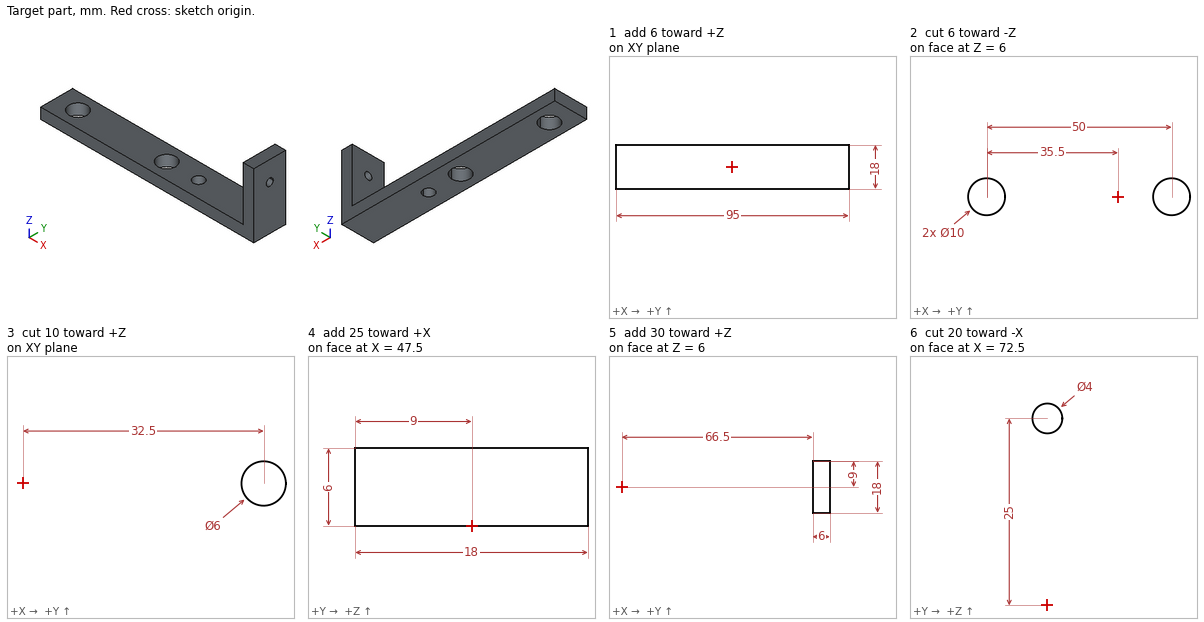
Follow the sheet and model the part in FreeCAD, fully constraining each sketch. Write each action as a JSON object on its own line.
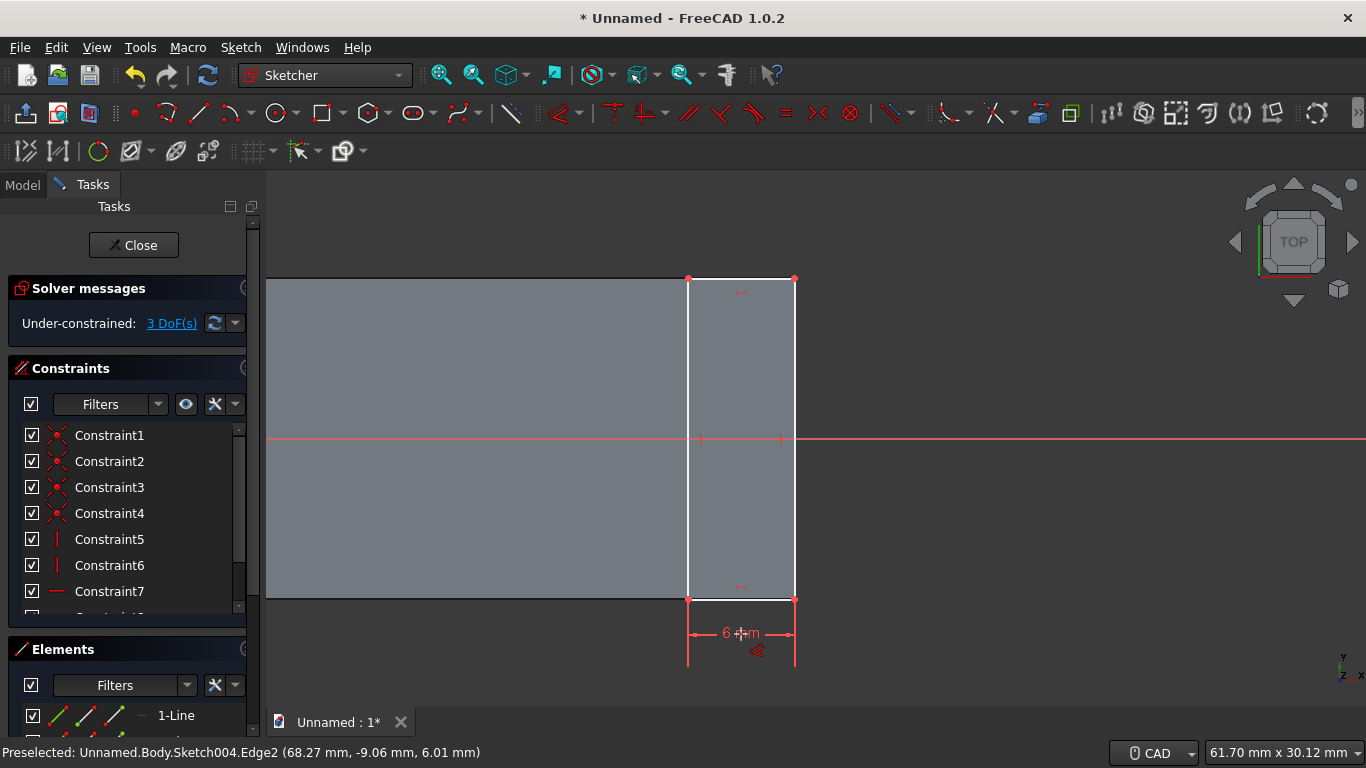
{"action": "left_click", "coordinate": [688, 375]}
{"action": "left_click", "coordinate": [654, 366]}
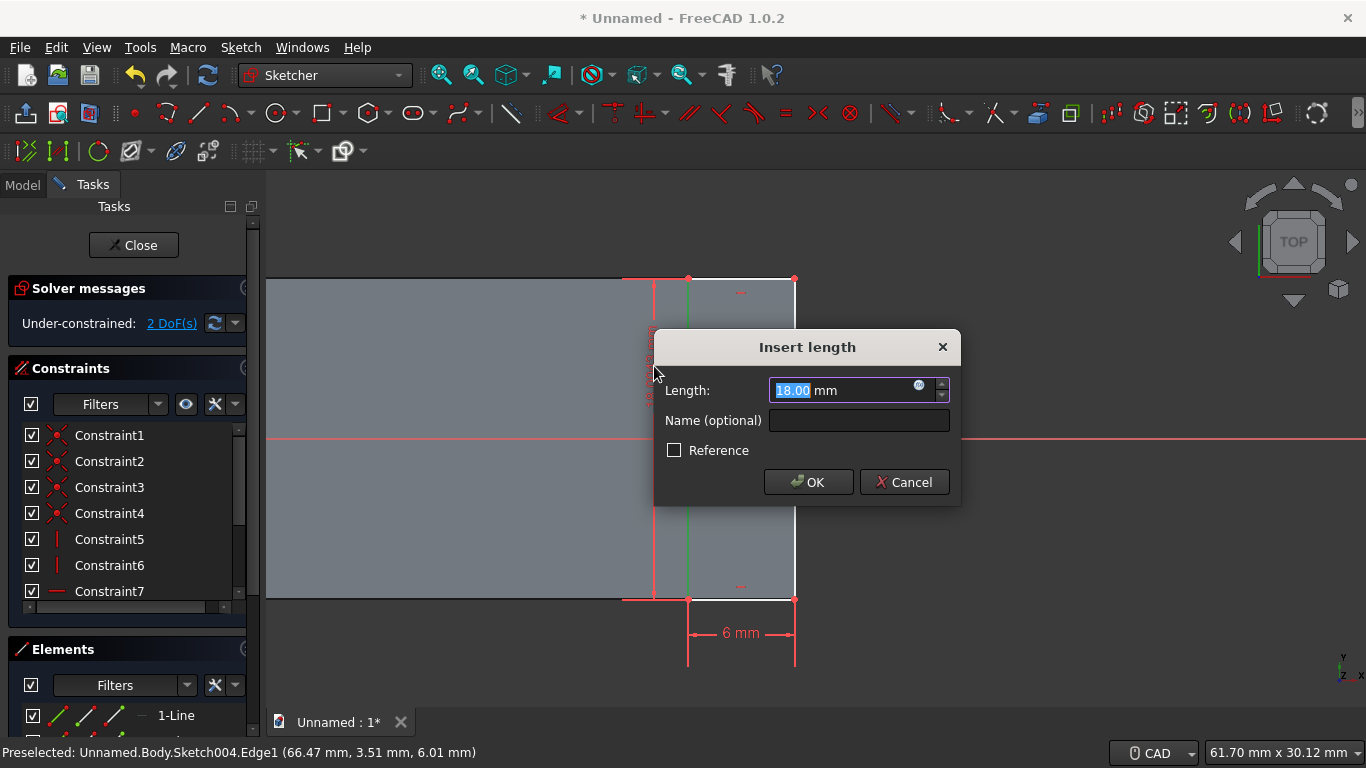
{"action": "type", "text": "18"}
{"action": "key", "text": "Return"}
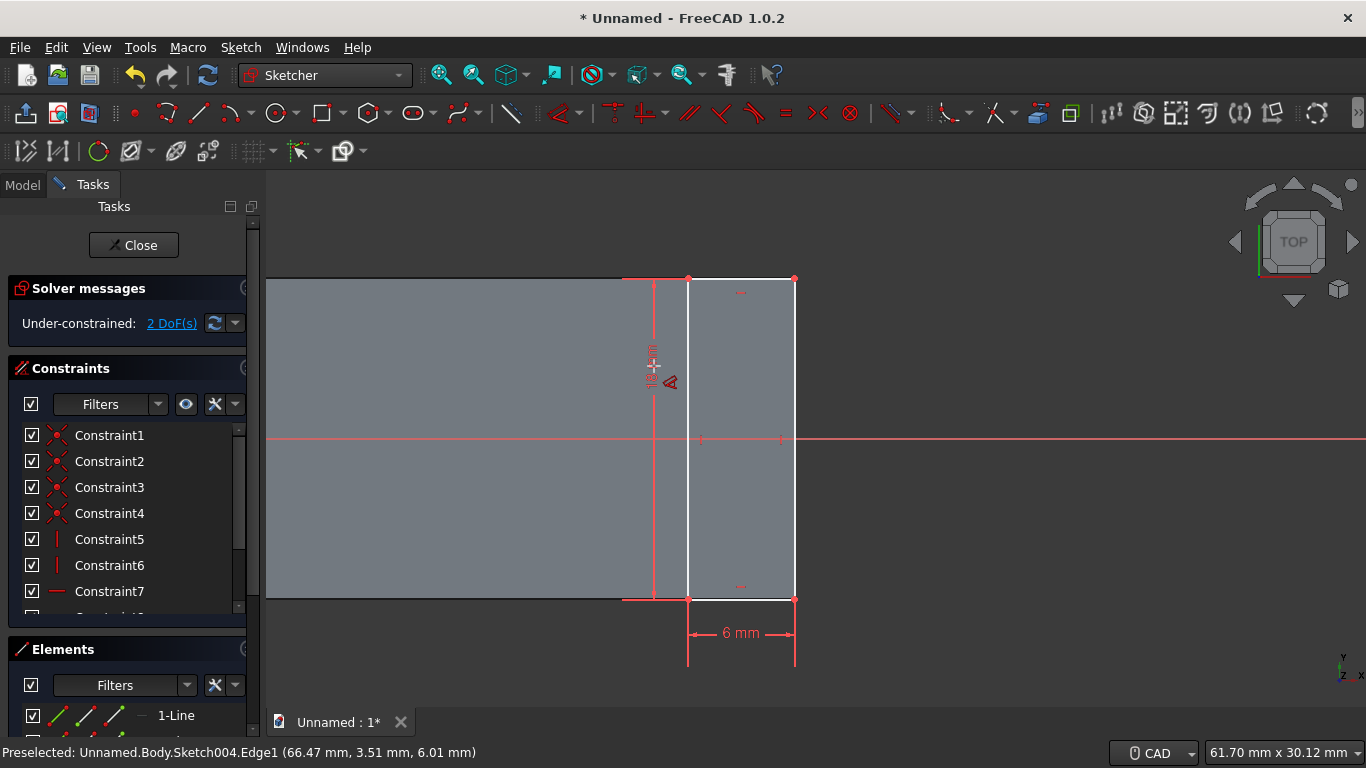
{"action": "left_click", "coordinate": [688, 279]}
{"action": "left_click", "coordinate": [722, 322]}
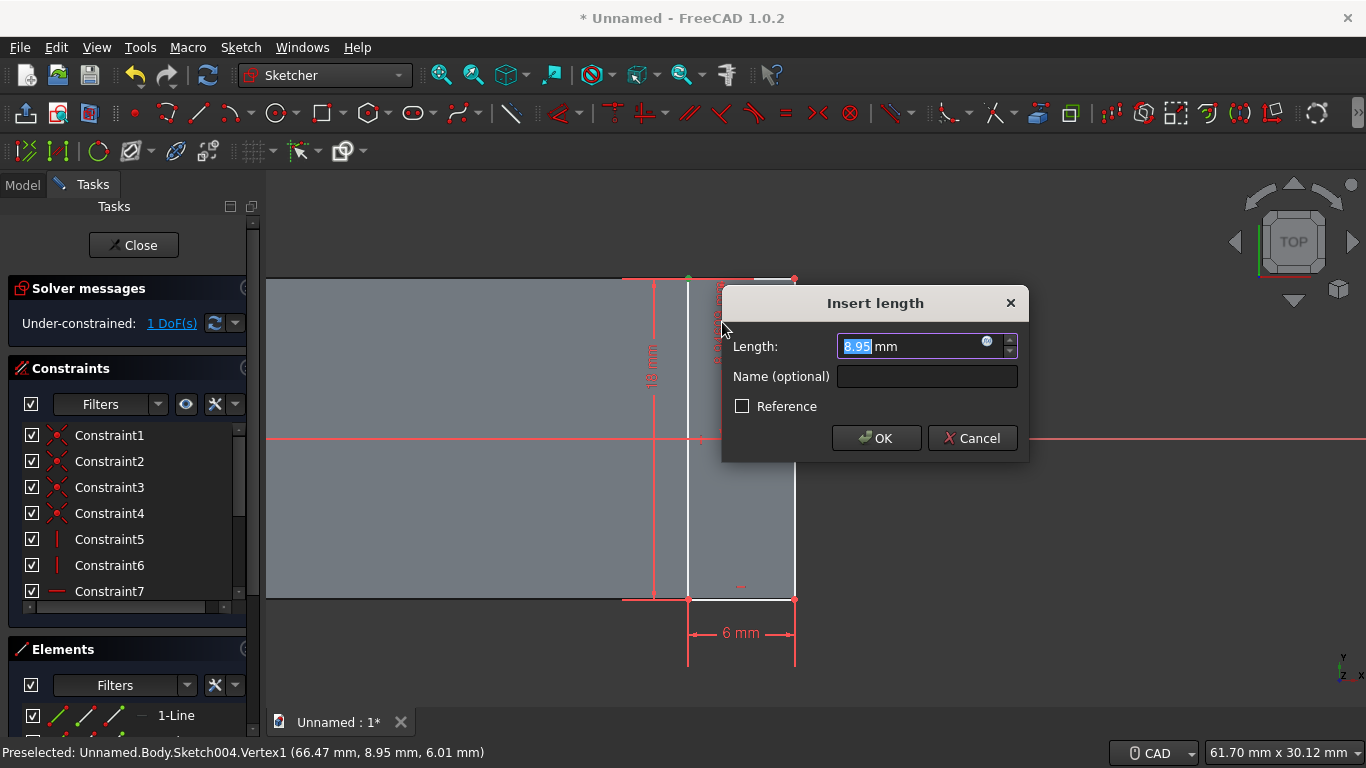
{"action": "type", "text": "9"}
{"action": "key", "text": "Return"}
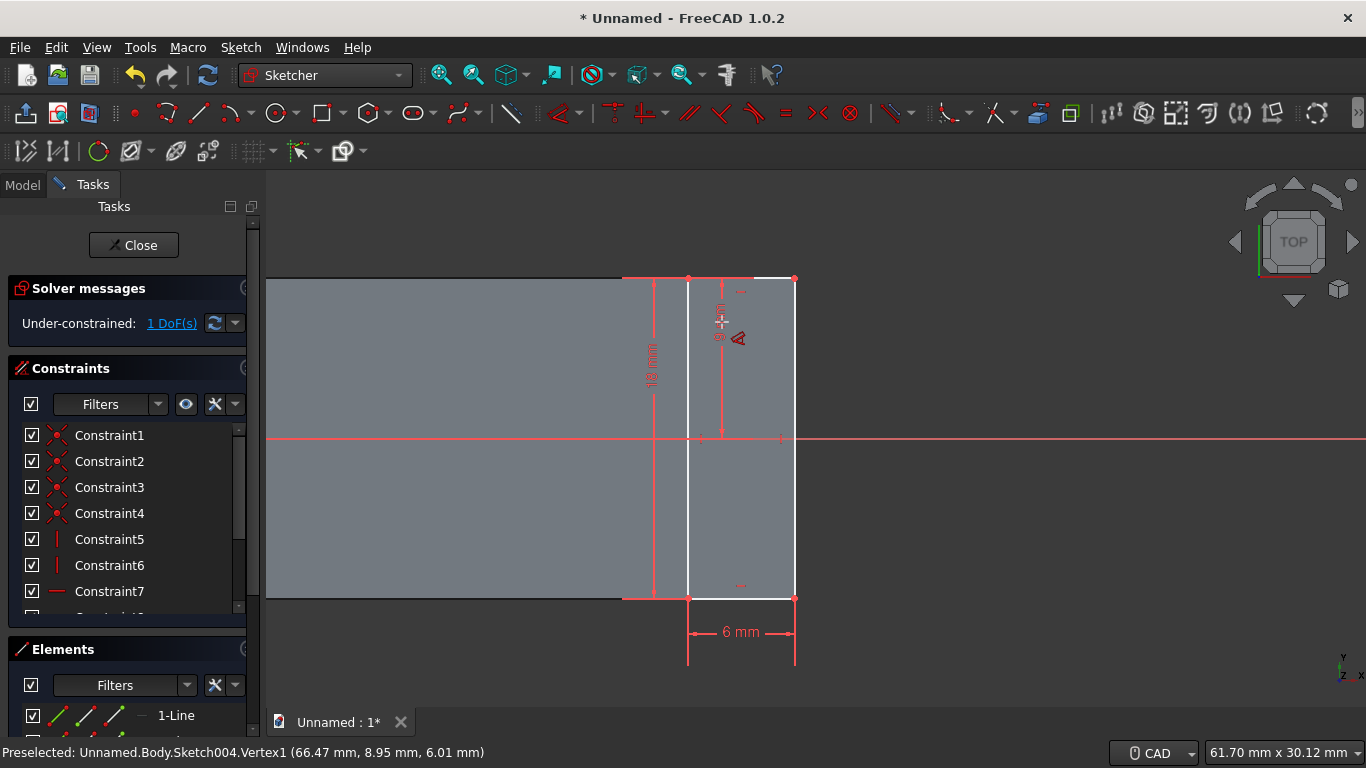
{"action": "left_click", "coordinate": [688, 278]}
{"action": "left_click", "coordinate": [491, 244]}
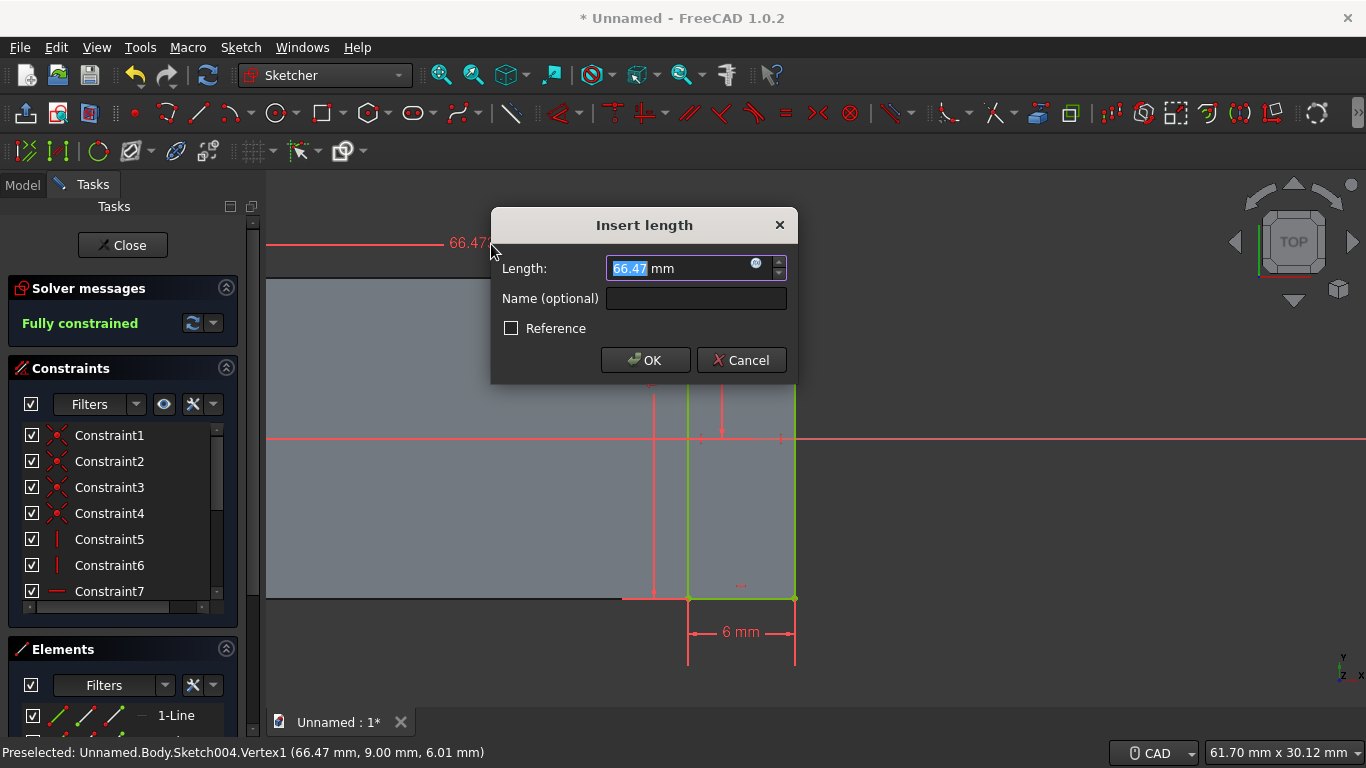
{"action": "type", "text": "66.5"}
{"action": "key", "text": "Return"}
{"action": "key", "text": "Escape"}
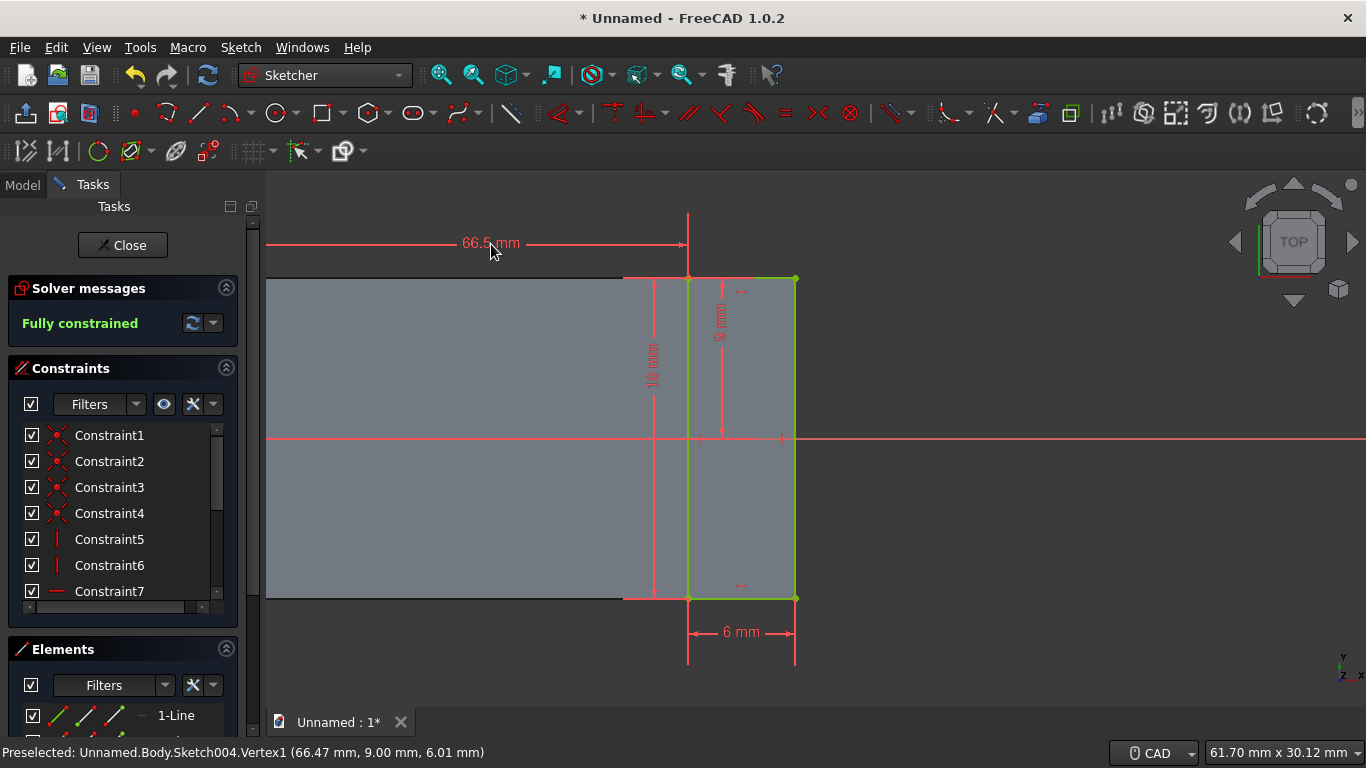
{"action": "left_click", "coordinate": [123, 245]}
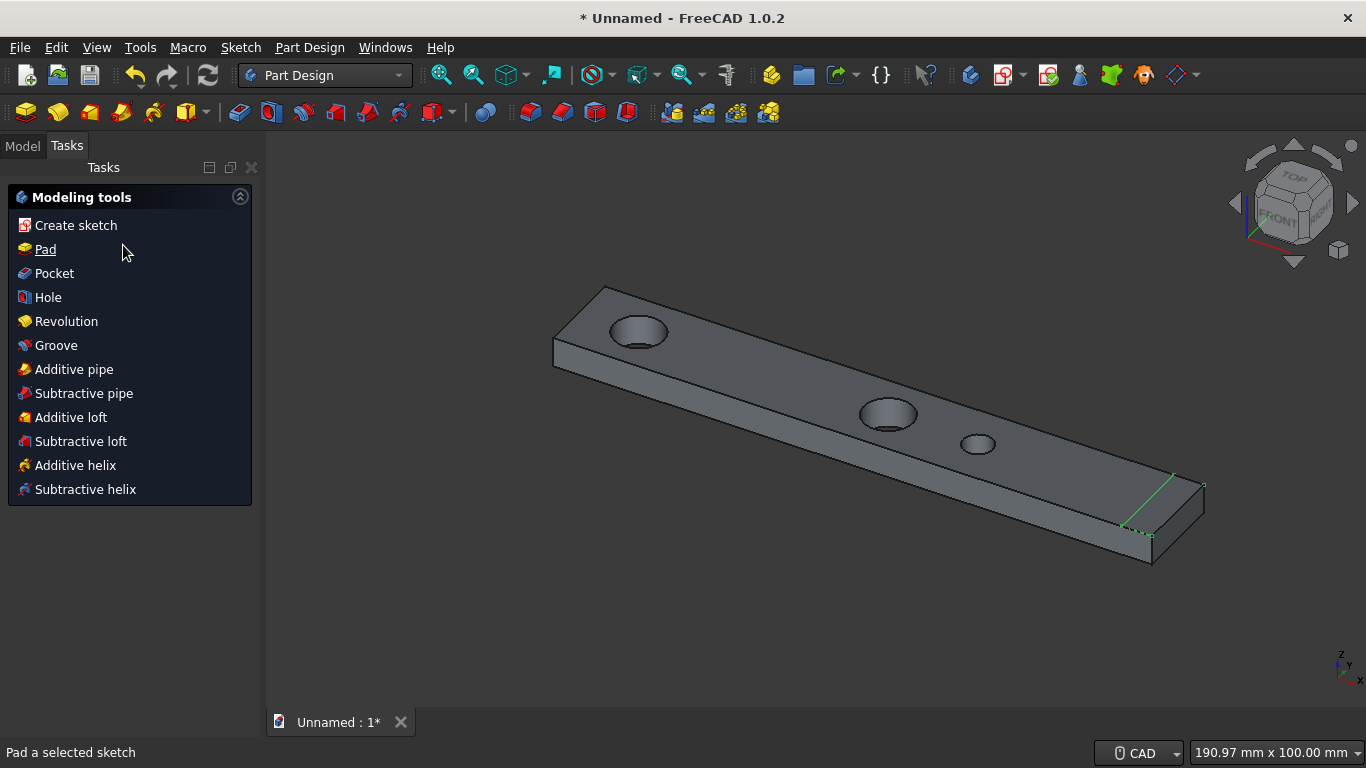
{"action": "left_click", "coordinate": [26, 112]}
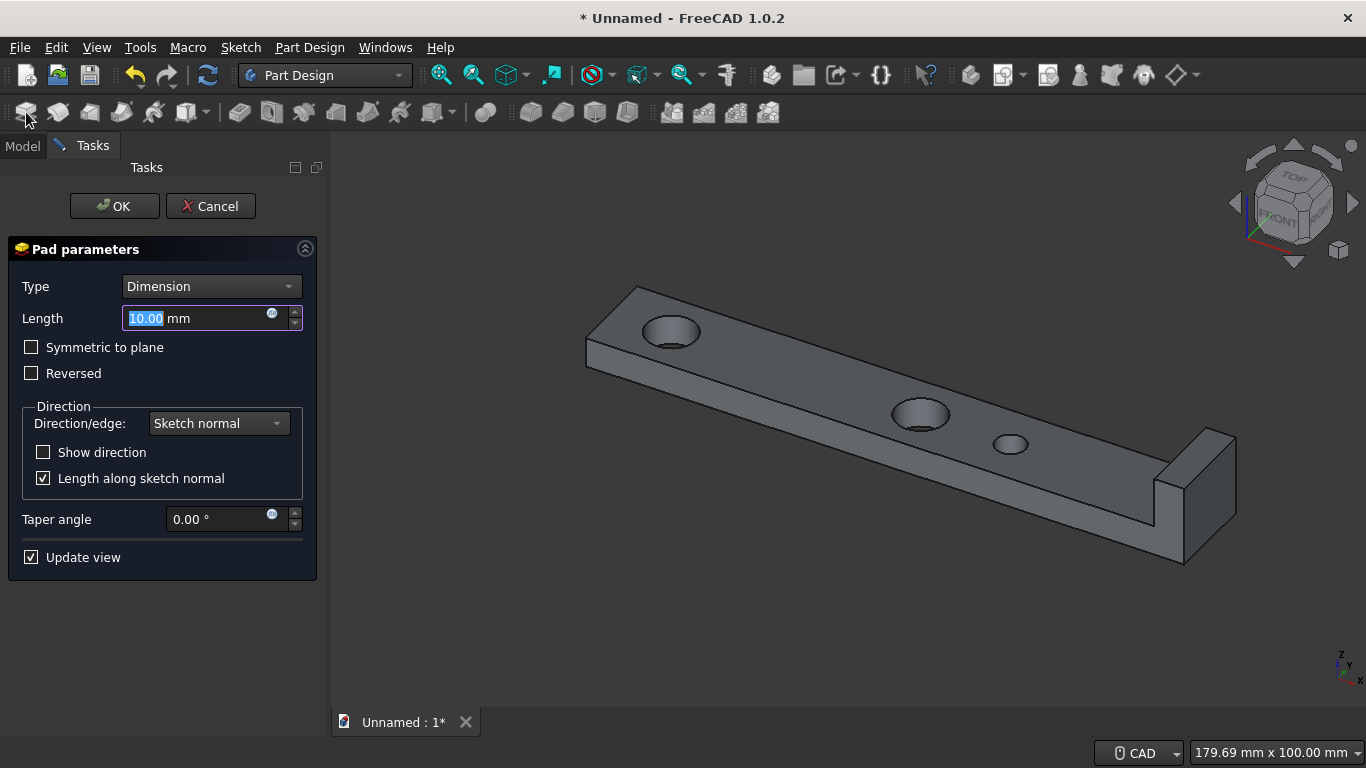
{"action": "type", "text": "30"}
{"action": "key", "text": "Tab"}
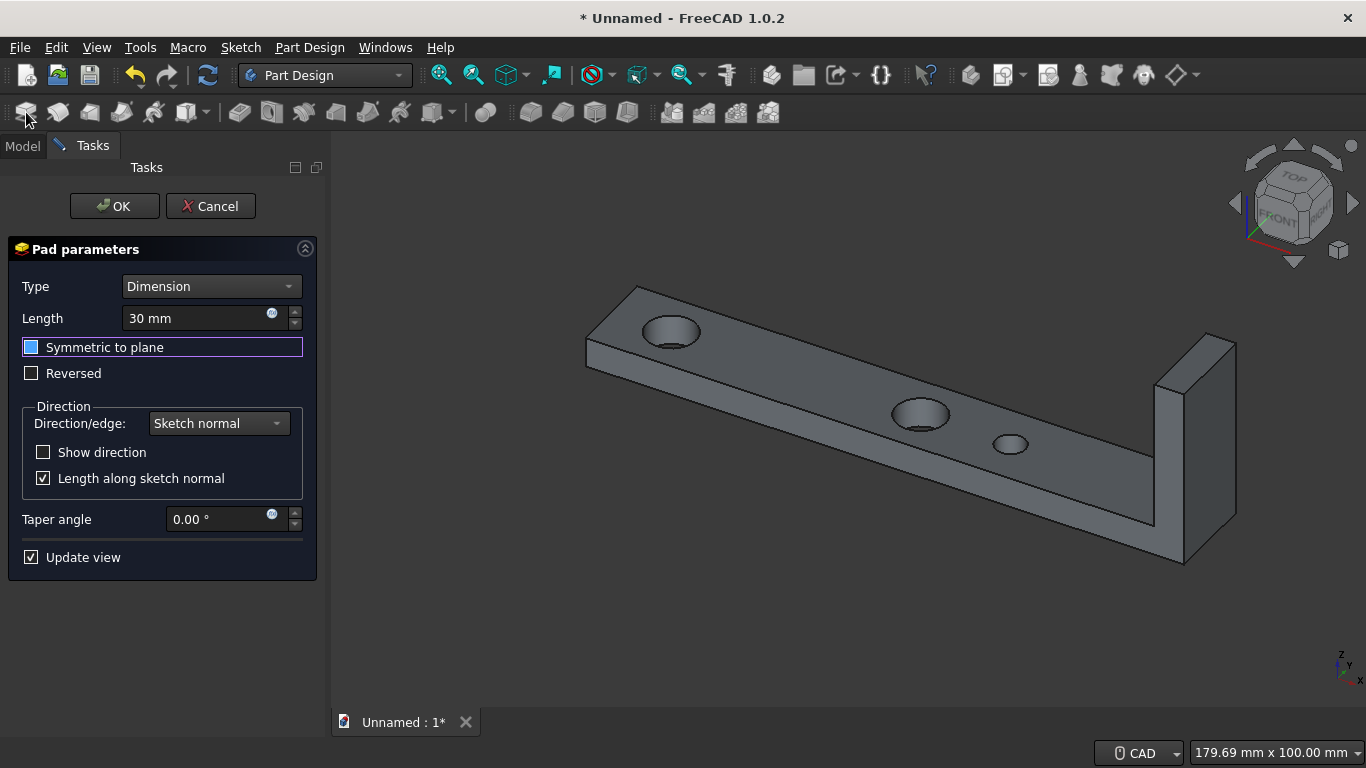
{"action": "left_click", "coordinate": [115, 206]}